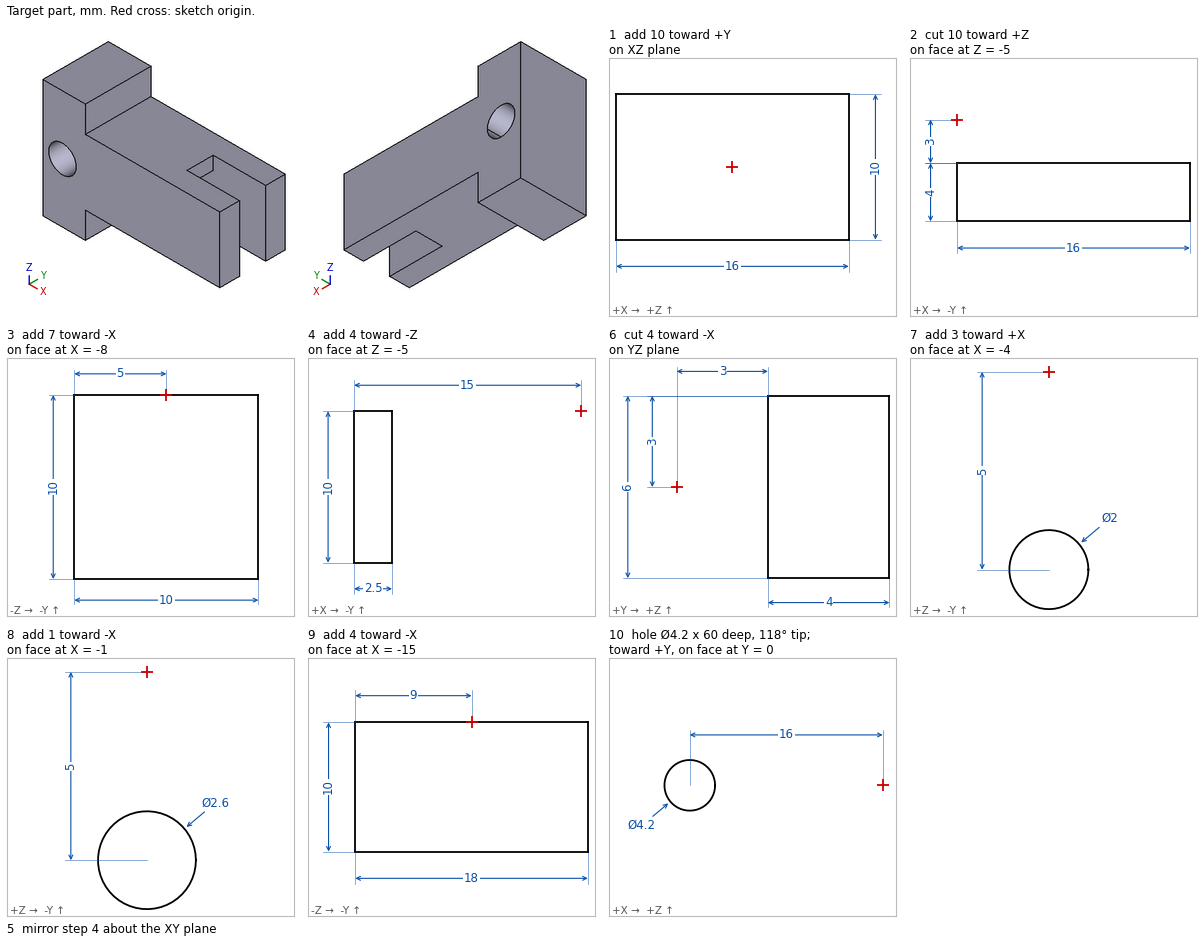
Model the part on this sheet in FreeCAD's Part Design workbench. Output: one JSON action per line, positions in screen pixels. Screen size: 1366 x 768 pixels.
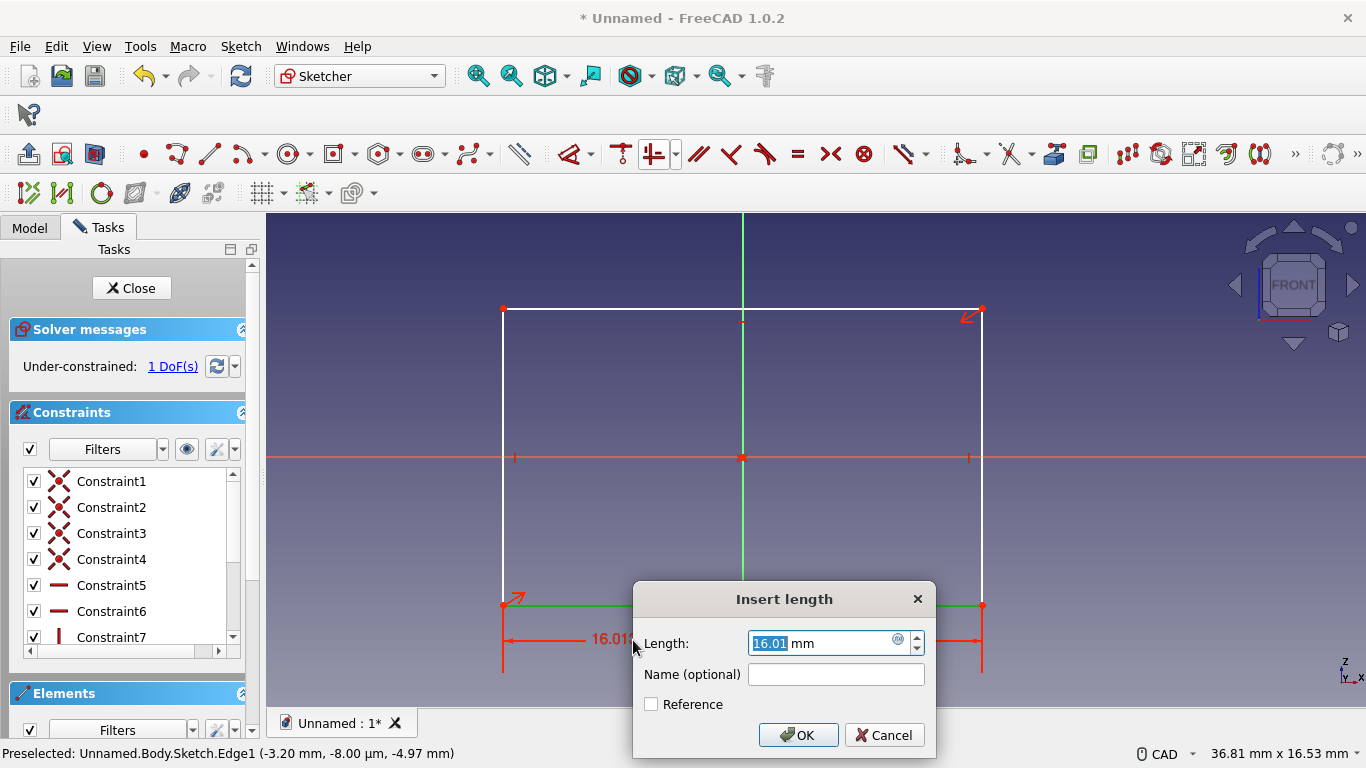
{"action": "type", "text": "16"}
{"action": "key", "text": "Return"}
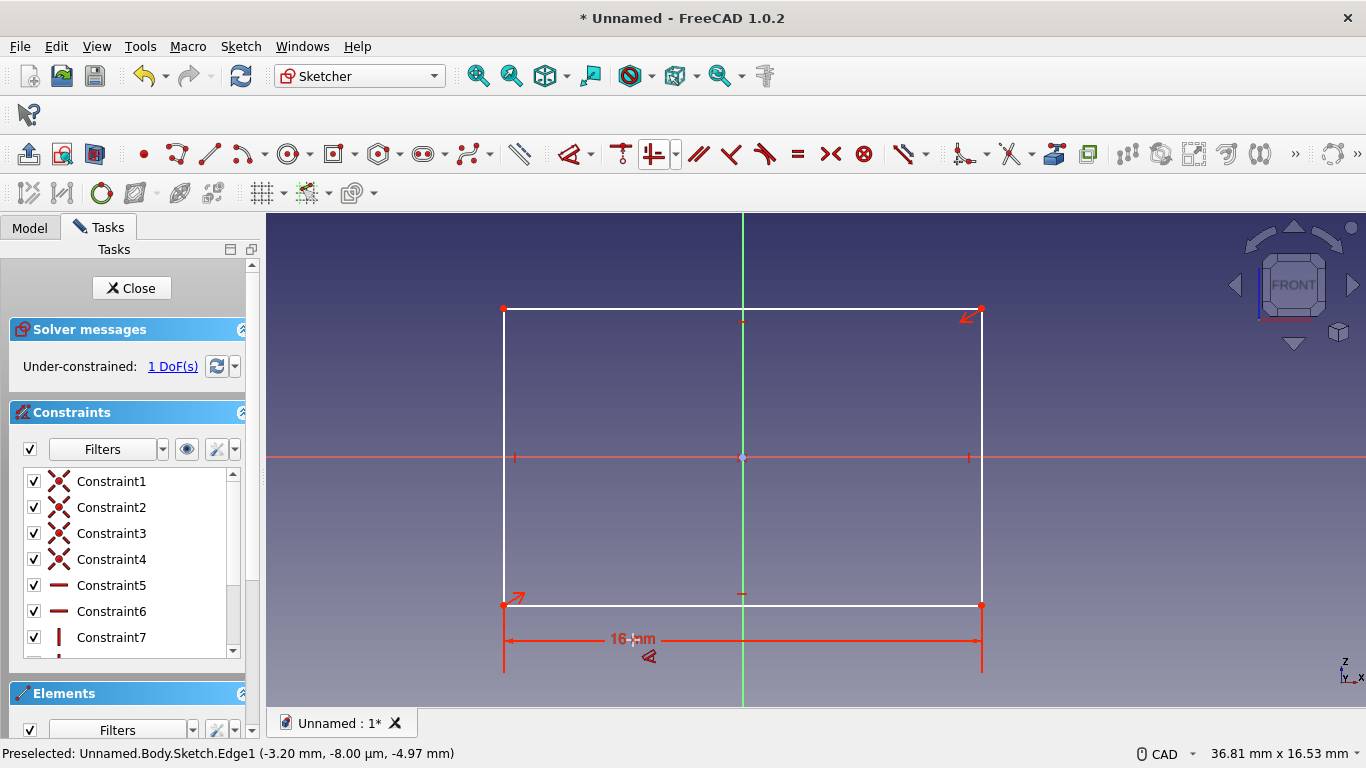
{"action": "left_click", "coordinate": [982, 517]}
{"action": "left_click", "coordinate": [1016, 389]}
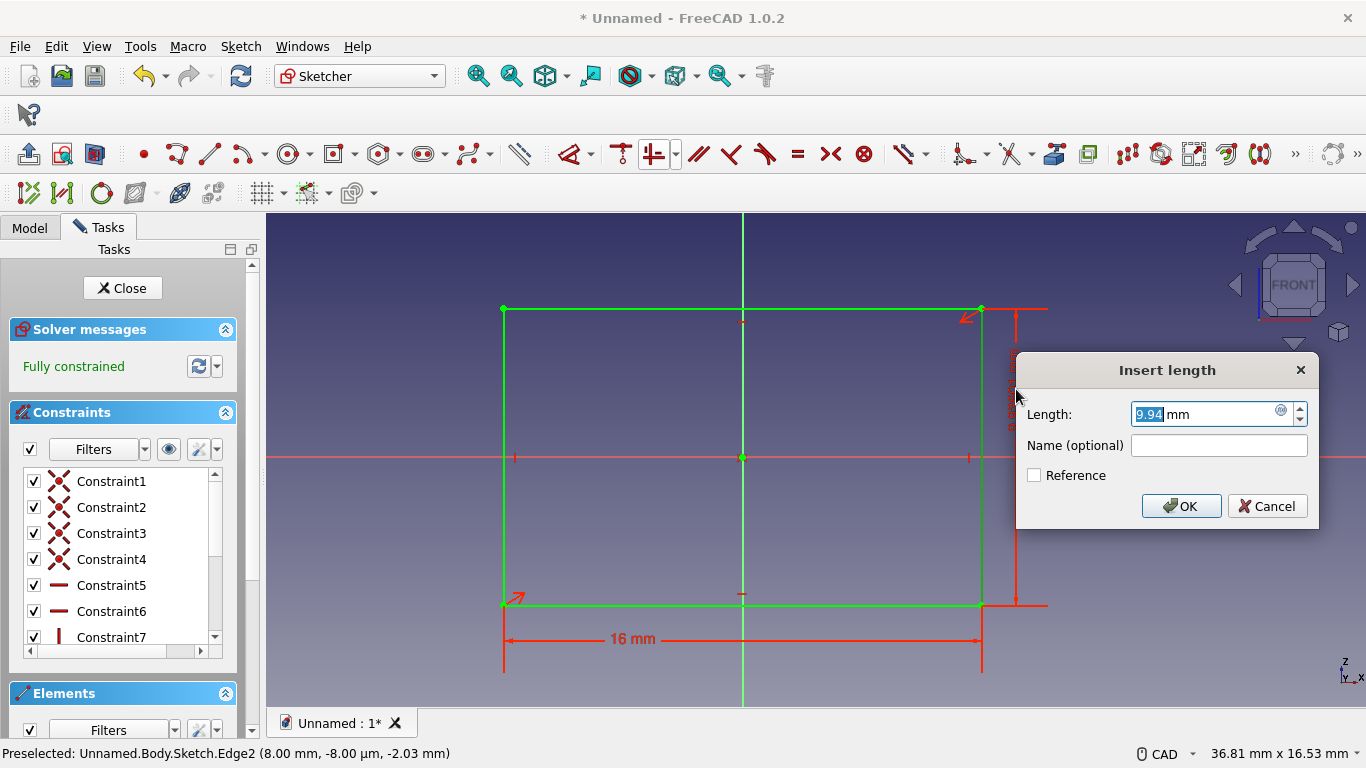
{"action": "type", "text": "10"}
{"action": "key", "text": "Return"}
{"action": "key", "text": "Escape"}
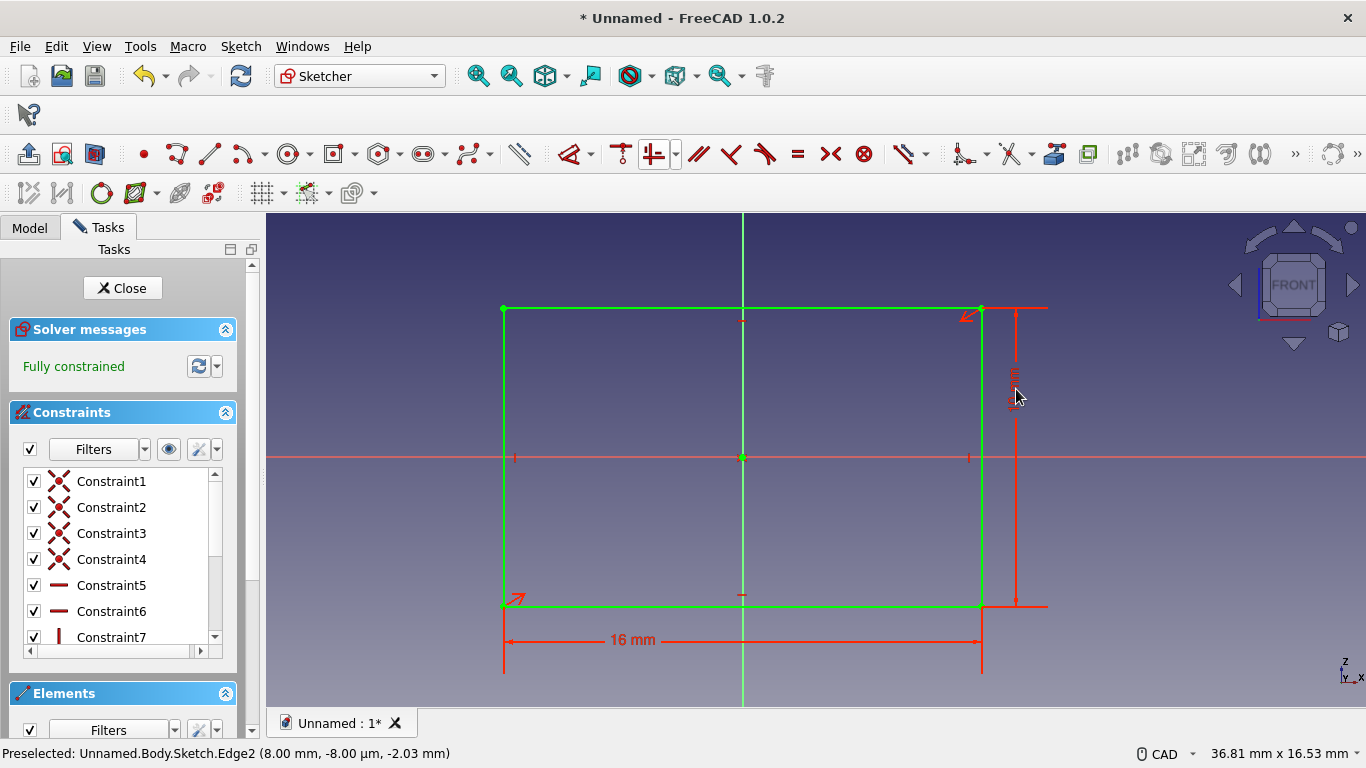
{"action": "left_click", "coordinate": [123, 288]}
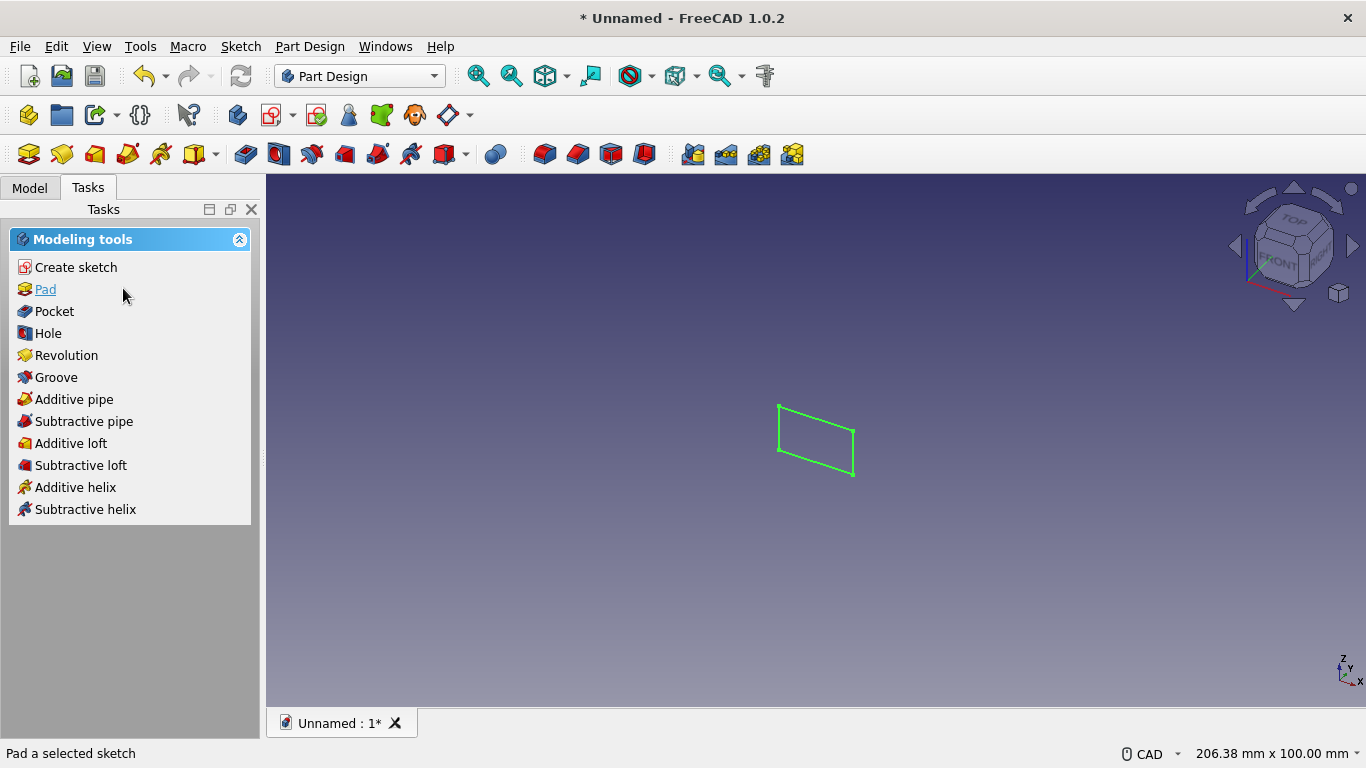
{"action": "left_click", "coordinate": [29, 154]}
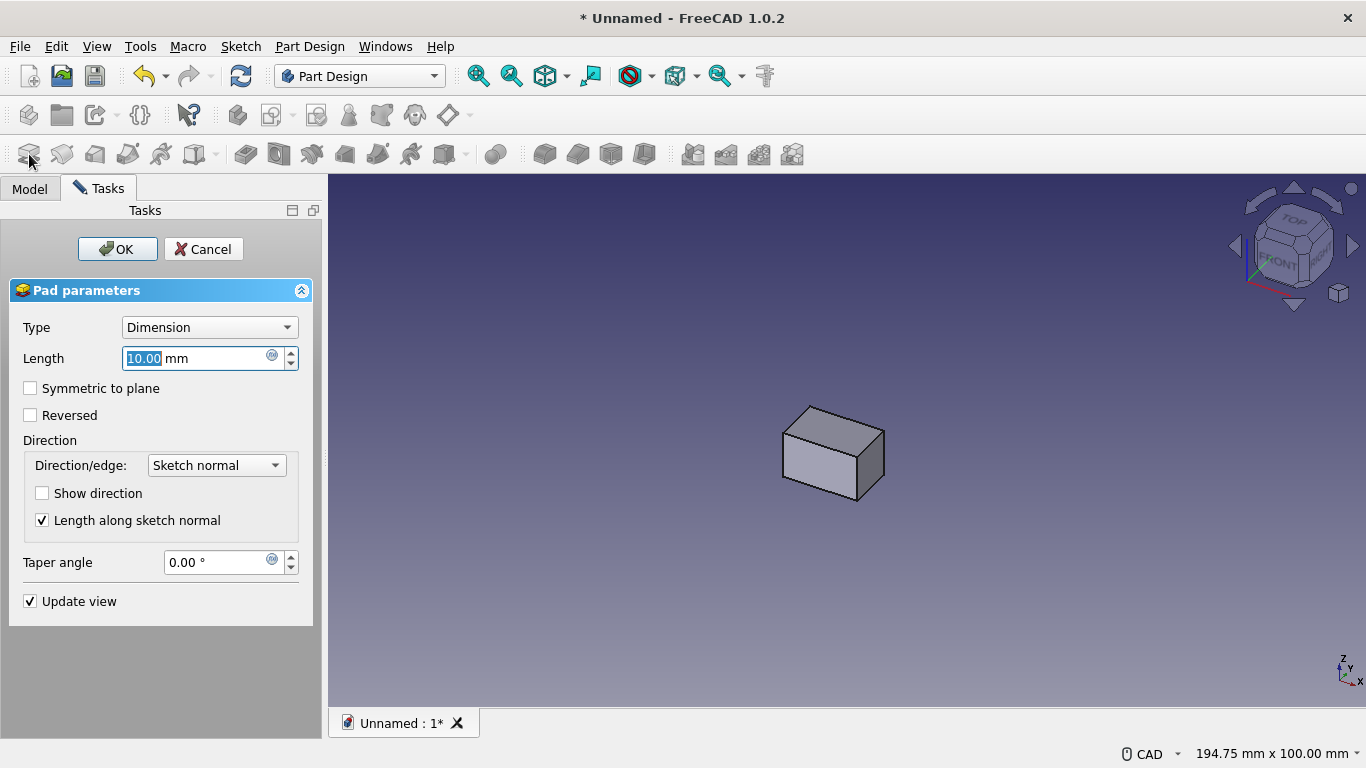
{"action": "type", "text": "10"}
{"action": "key", "text": "Tab"}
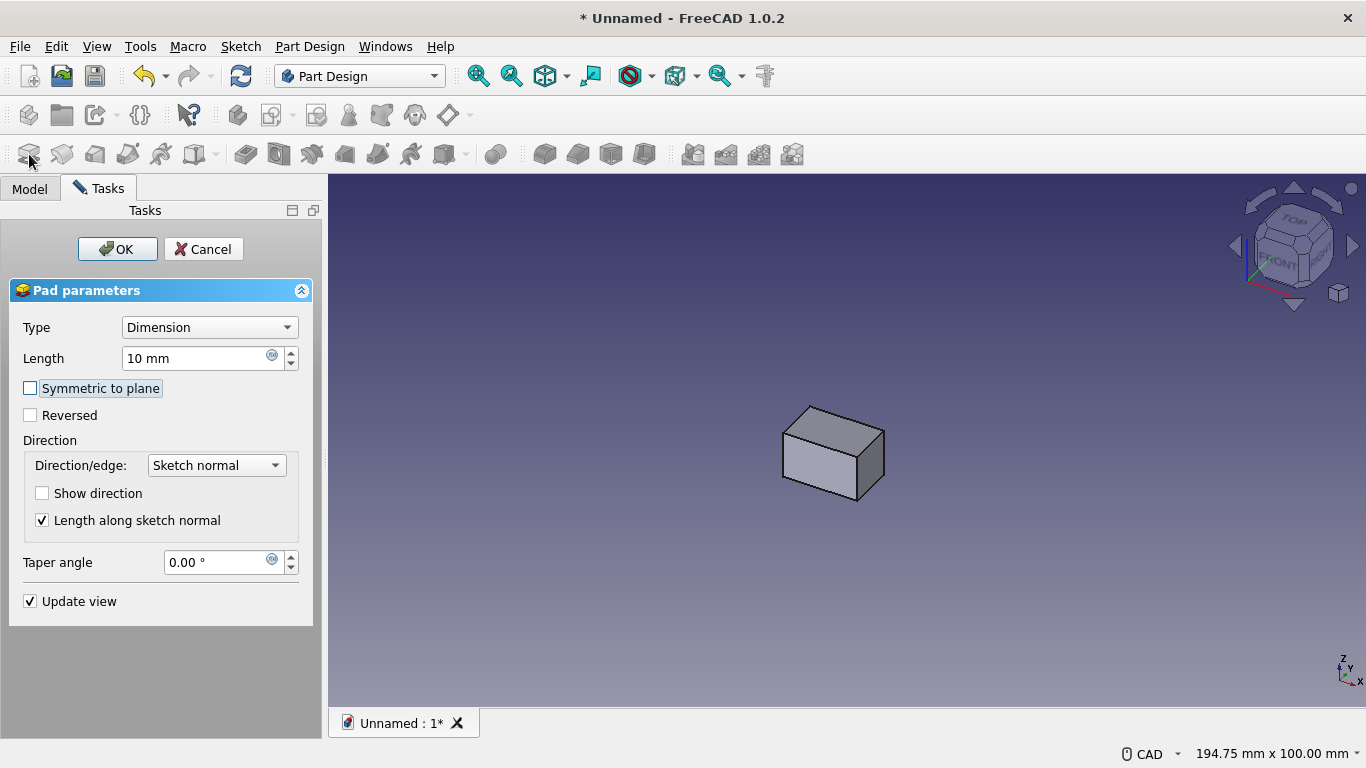
{"action": "left_click", "coordinate": [31, 415]}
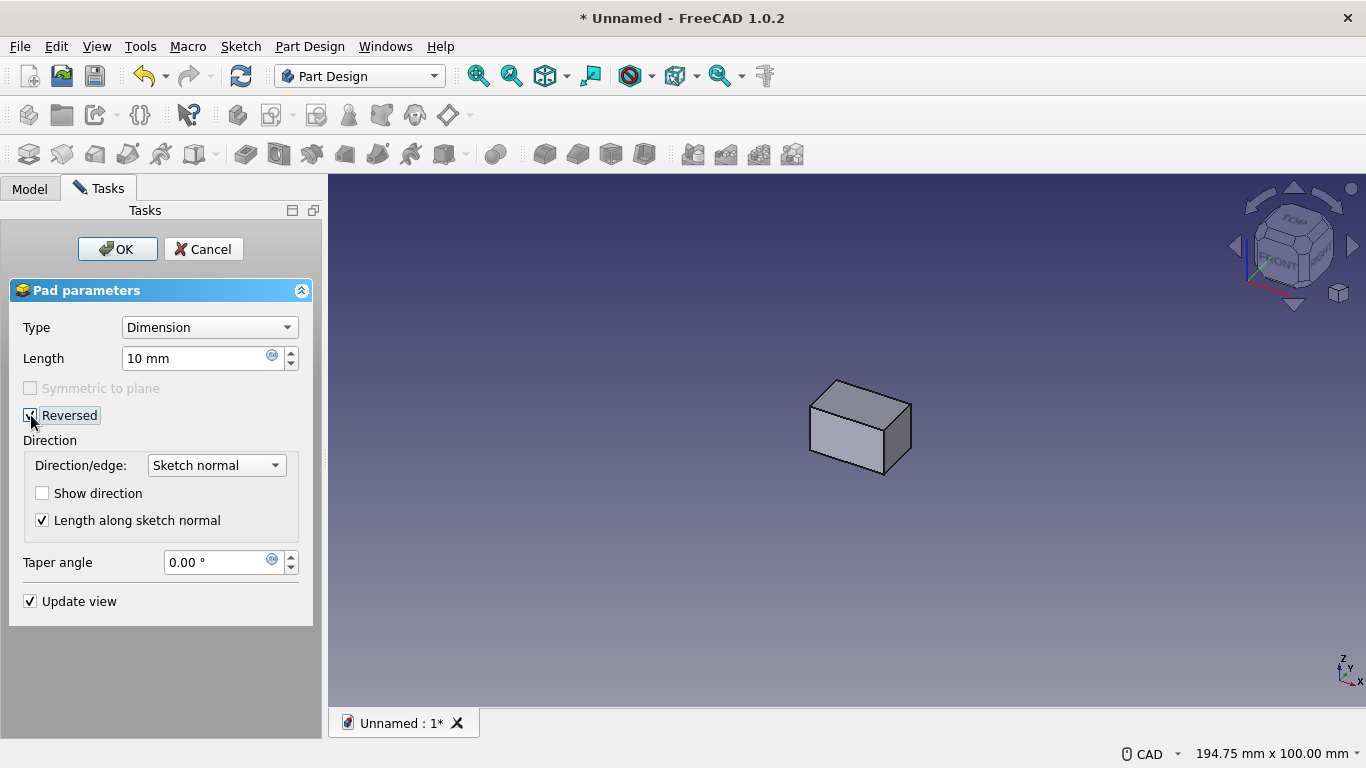
{"action": "left_click", "coordinate": [118, 249]}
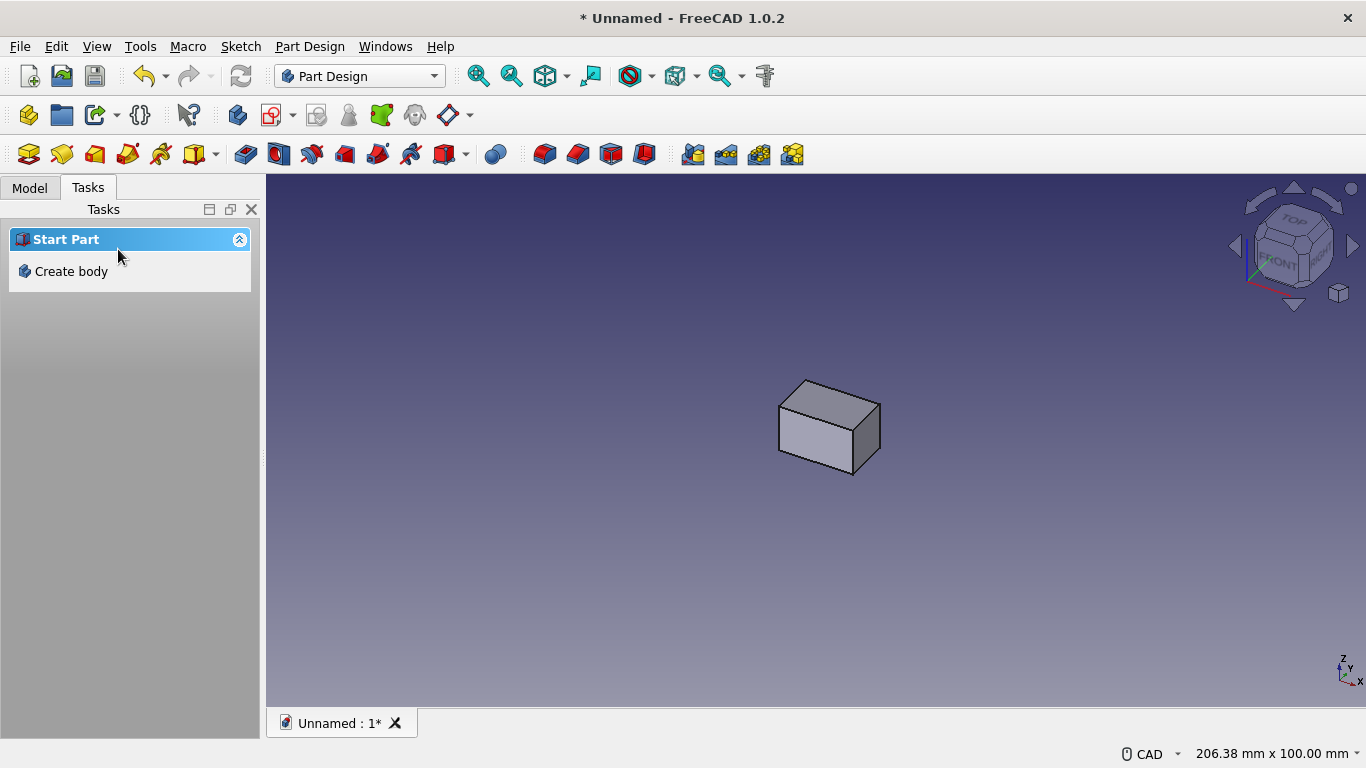
{"action": "left_click", "coordinate": [479, 76]}